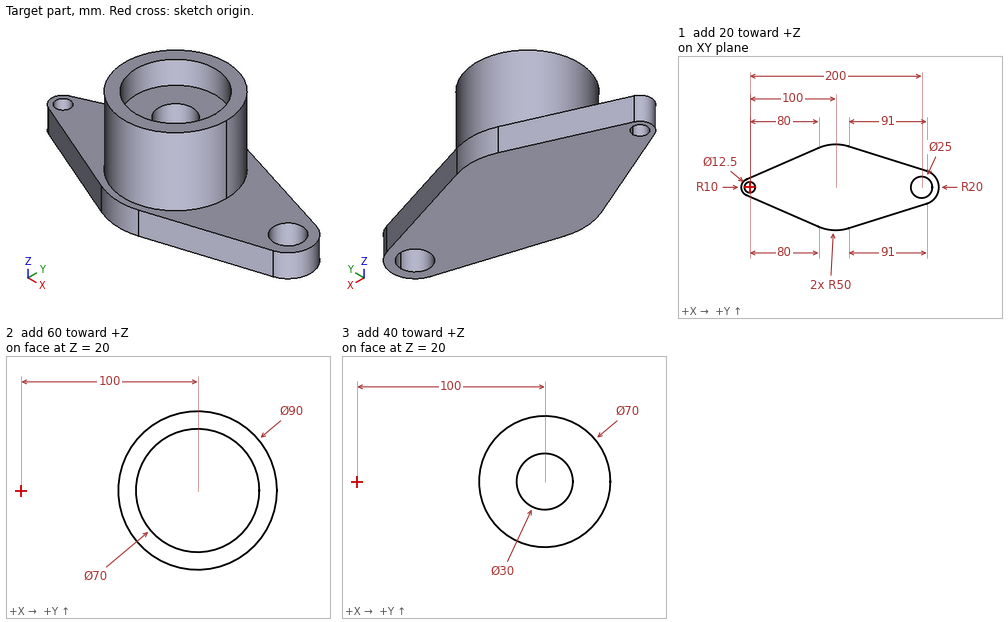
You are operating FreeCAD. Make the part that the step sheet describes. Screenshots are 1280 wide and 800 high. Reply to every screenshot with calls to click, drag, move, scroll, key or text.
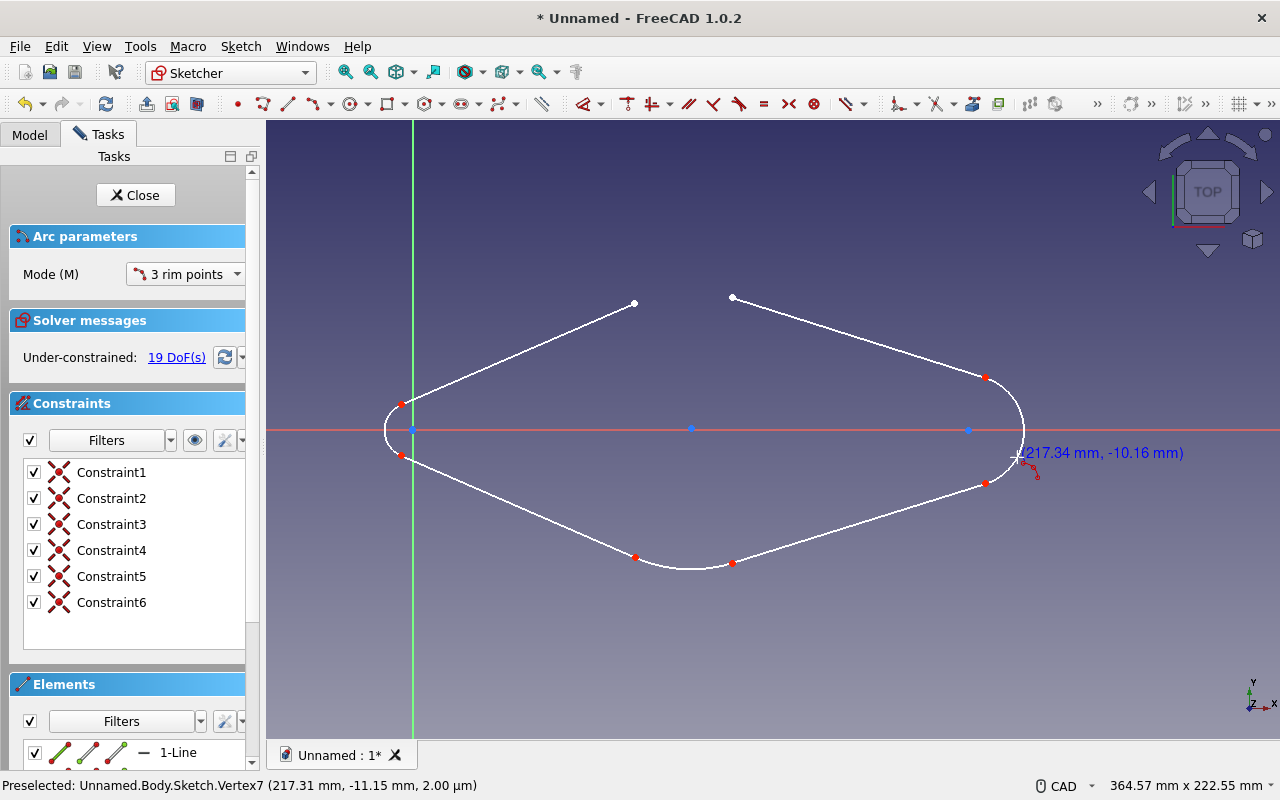
click(732, 298)
click(635, 304)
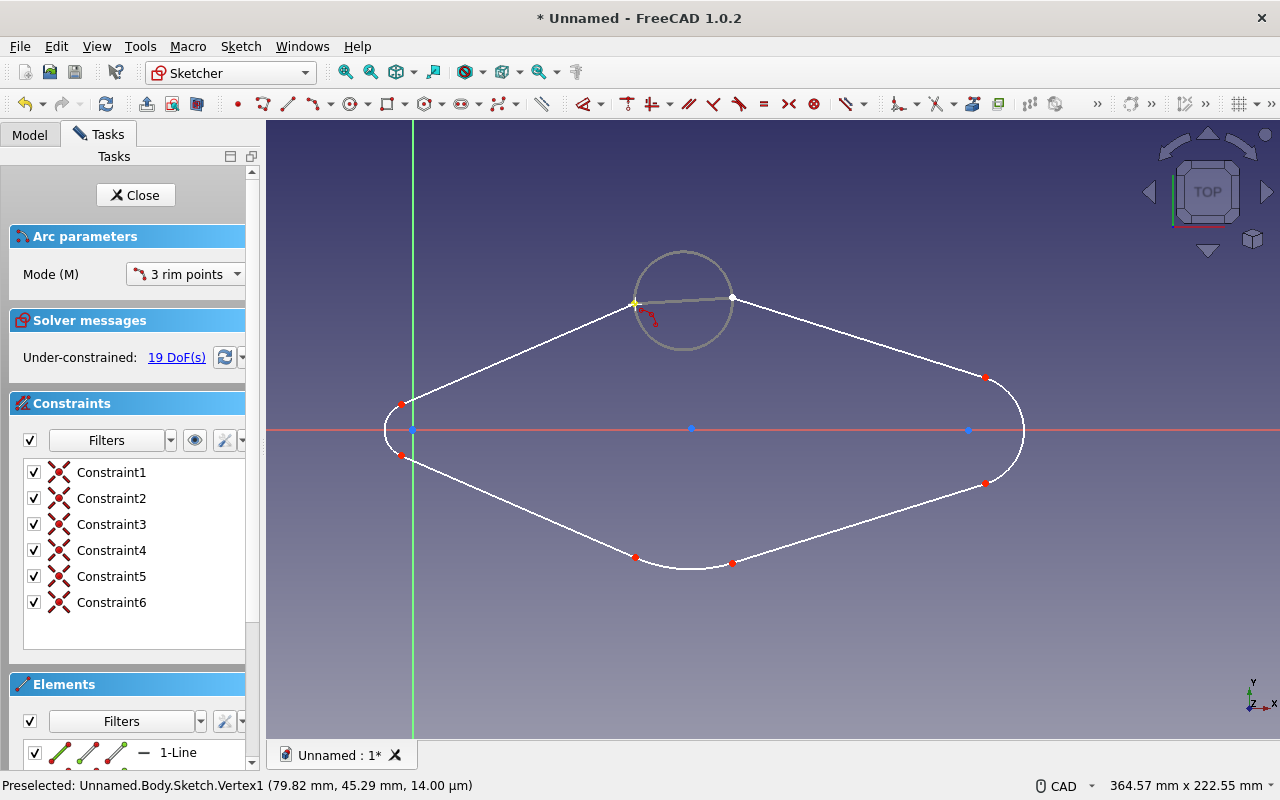
scroll(683, 291, up, 3)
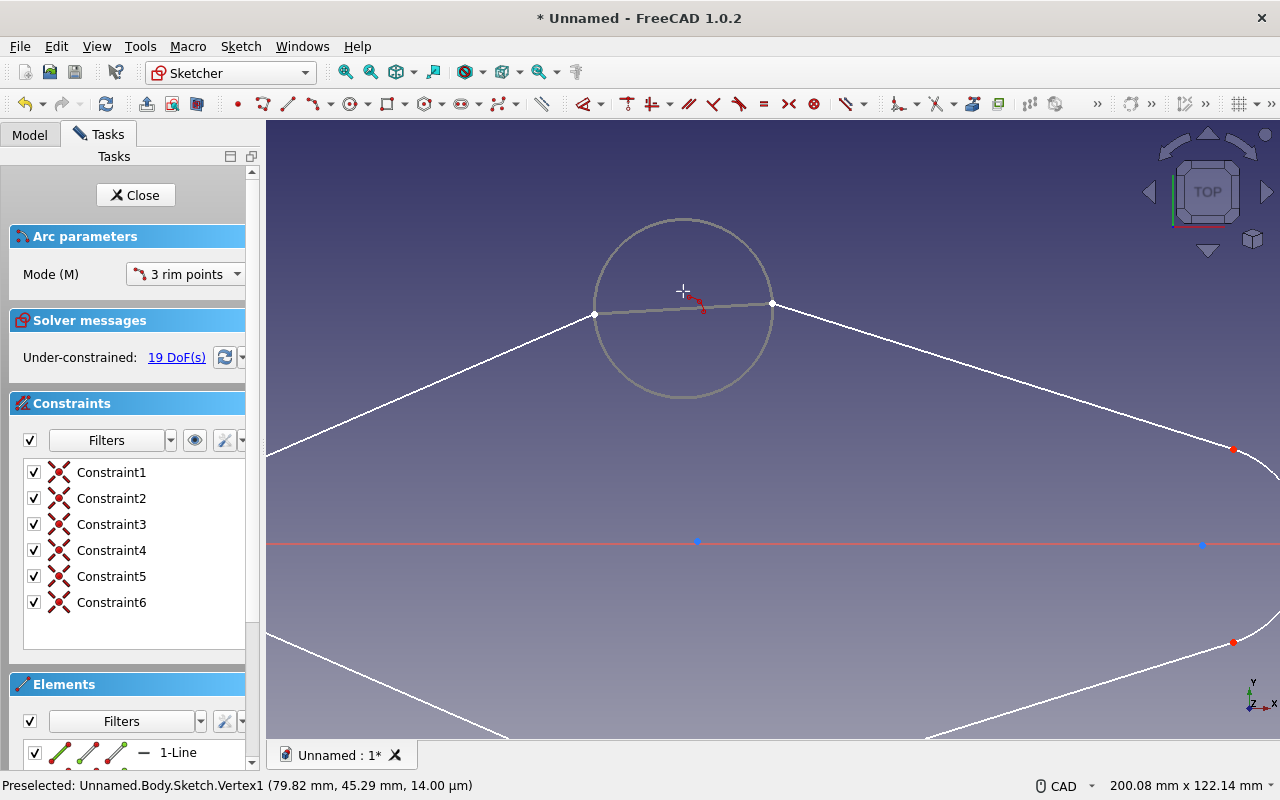
click(683, 291)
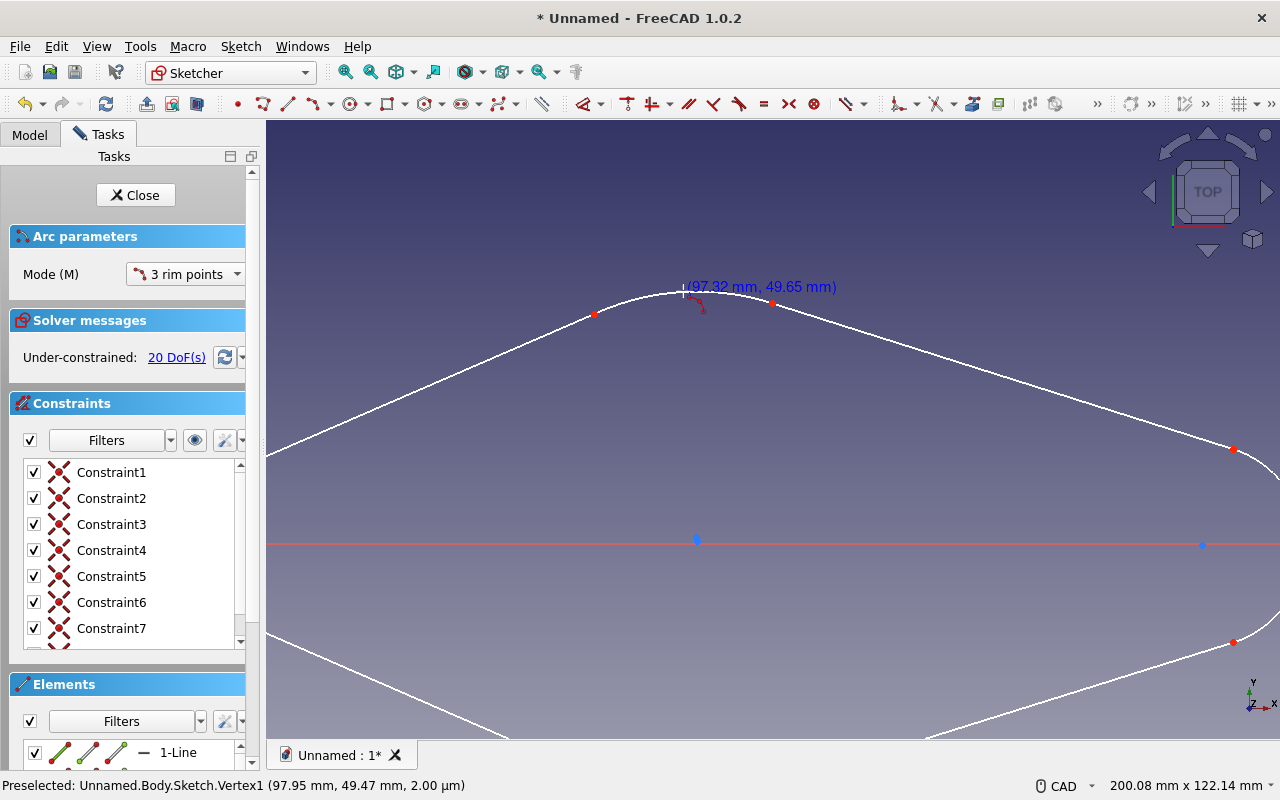
click(350, 104)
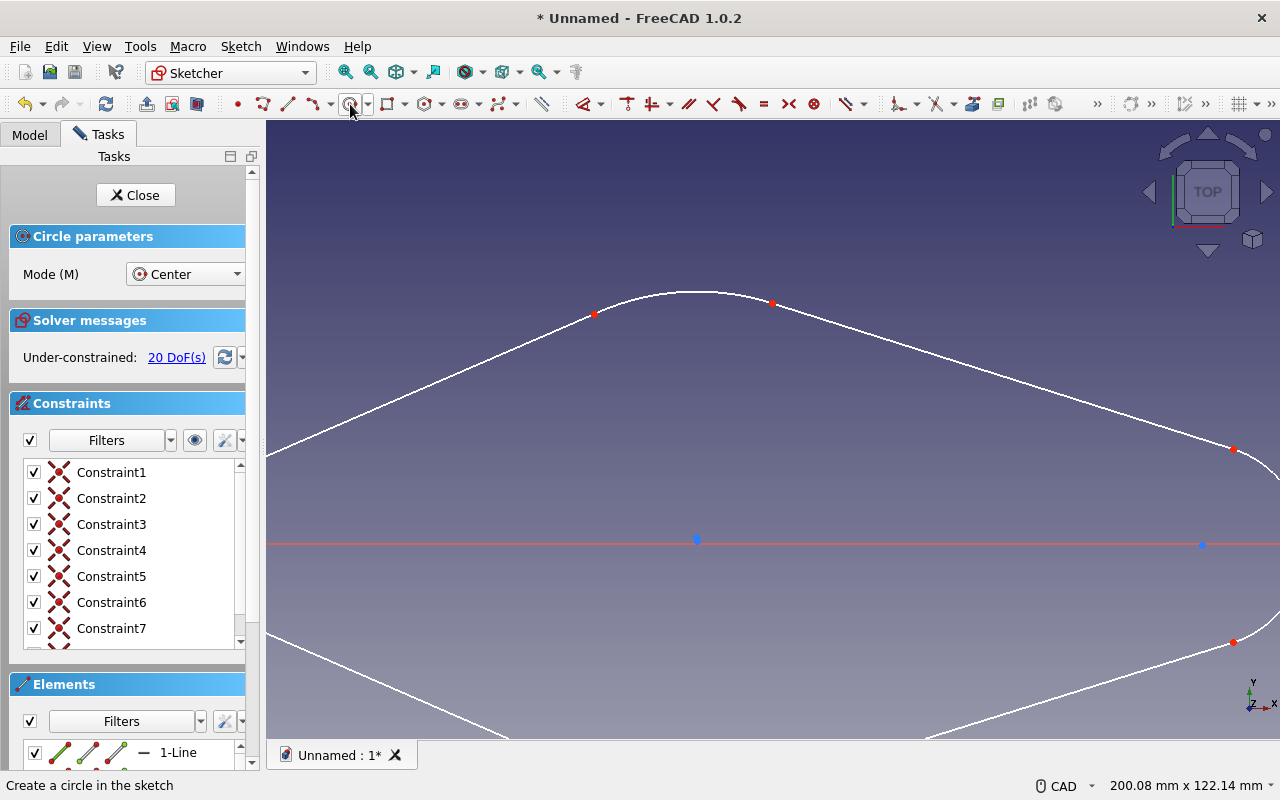
scroll(683, 291, down, 3)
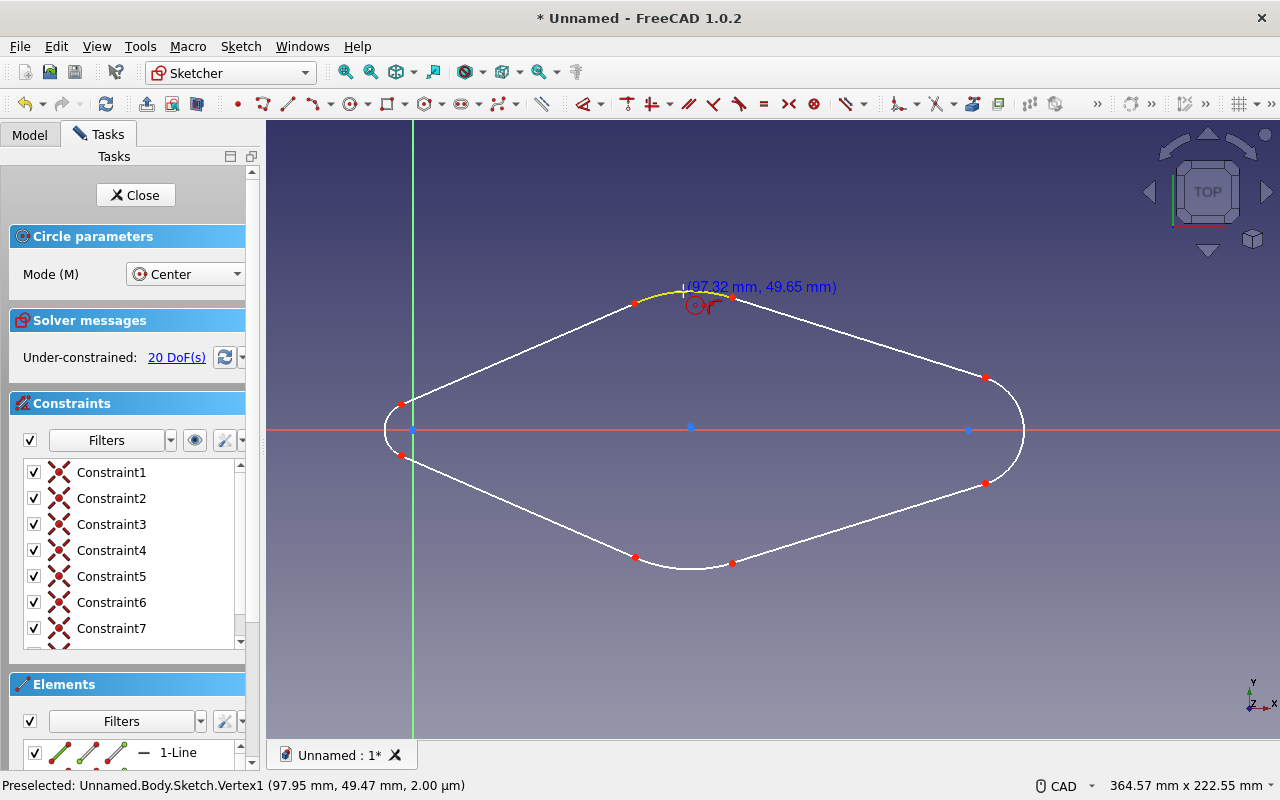
click(969, 430)
click(993, 405)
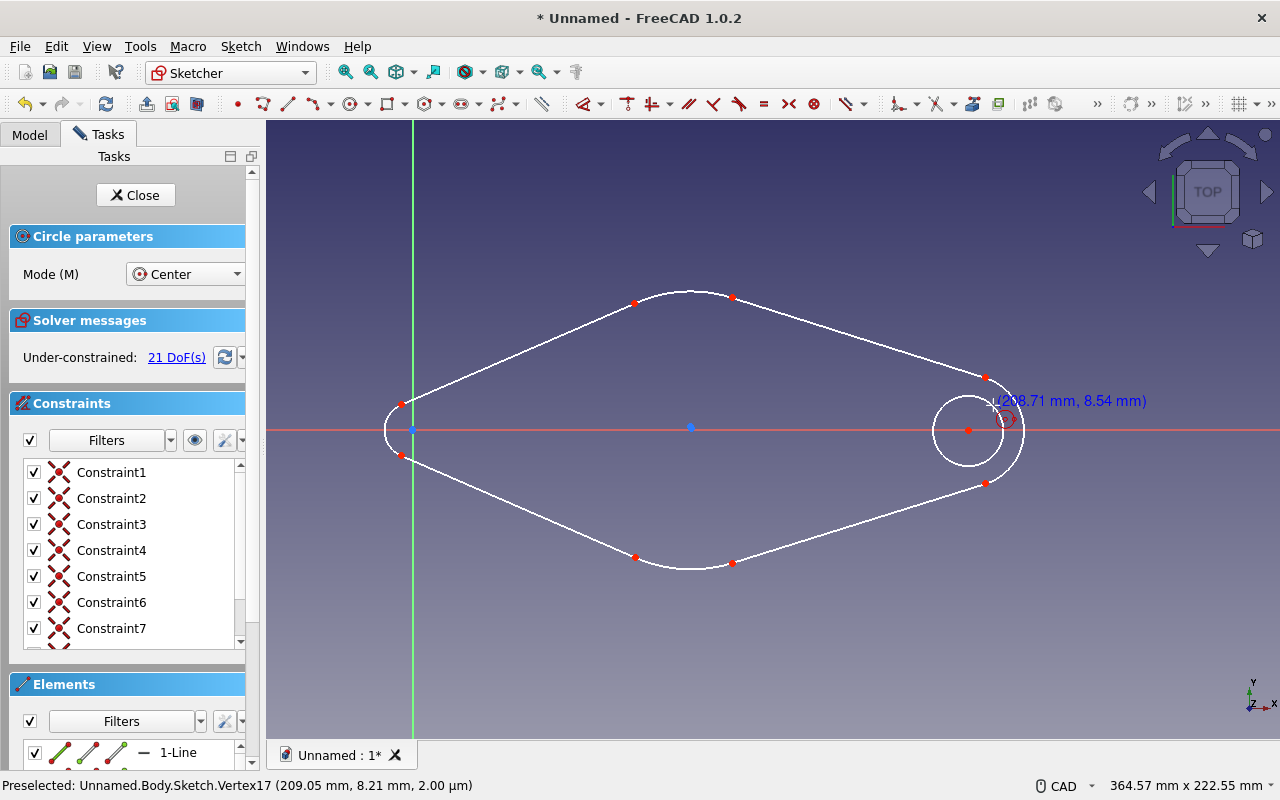
scroll(413, 430, up, 2)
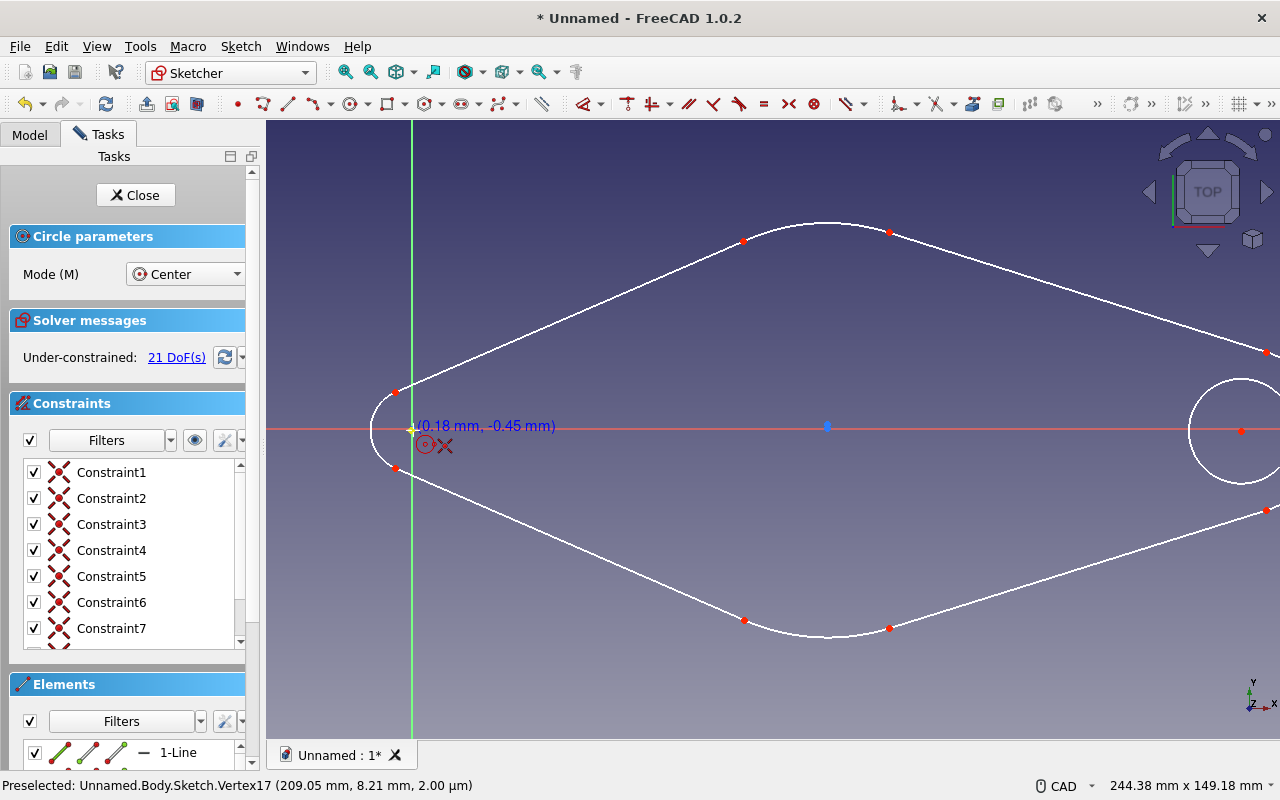
click(412, 429)
click(431, 411)
key(Escape)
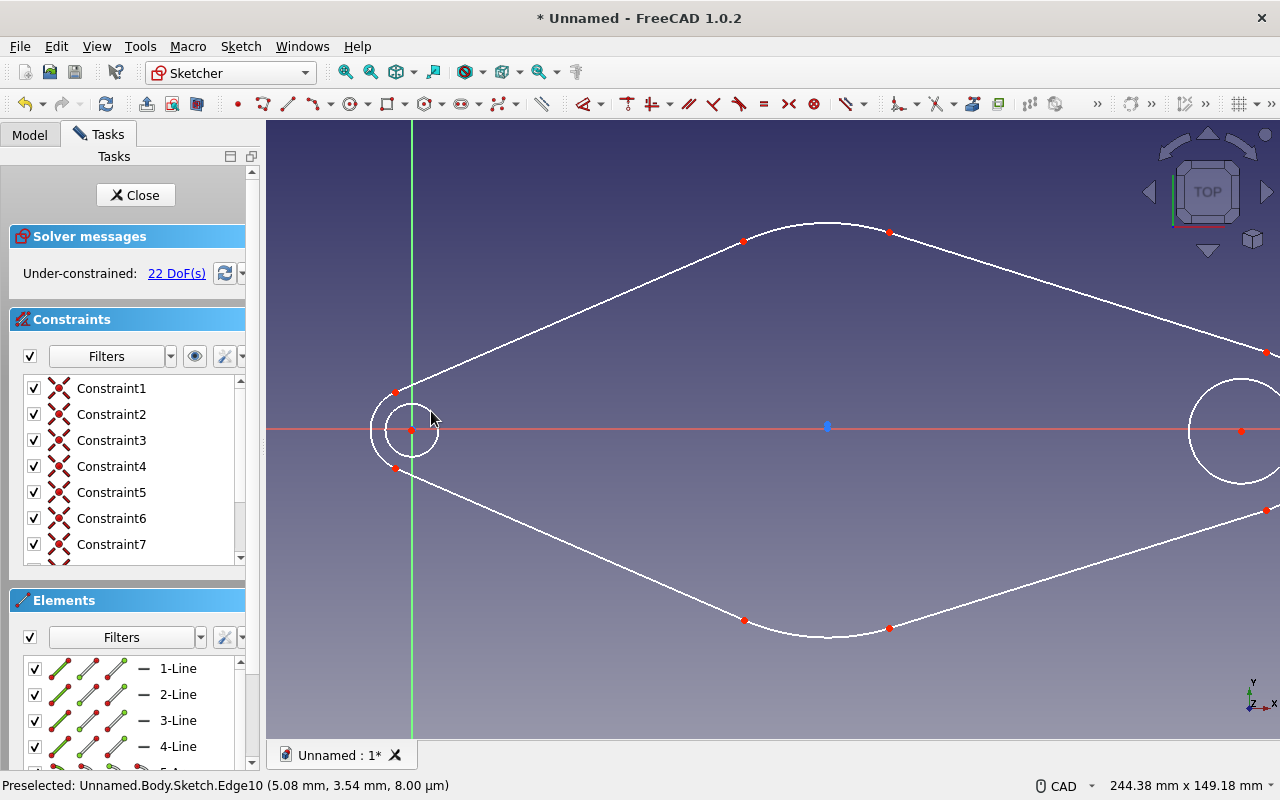
click(639, 287)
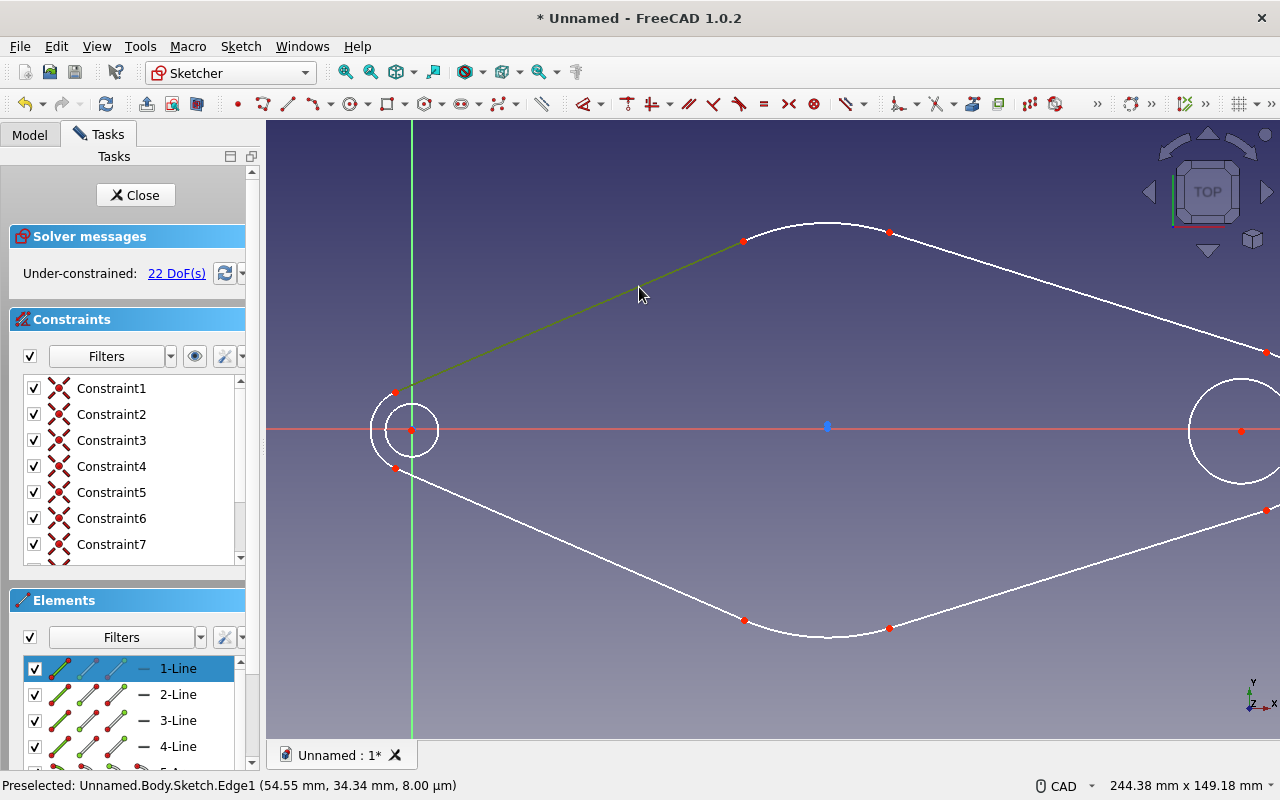
click(375, 412)